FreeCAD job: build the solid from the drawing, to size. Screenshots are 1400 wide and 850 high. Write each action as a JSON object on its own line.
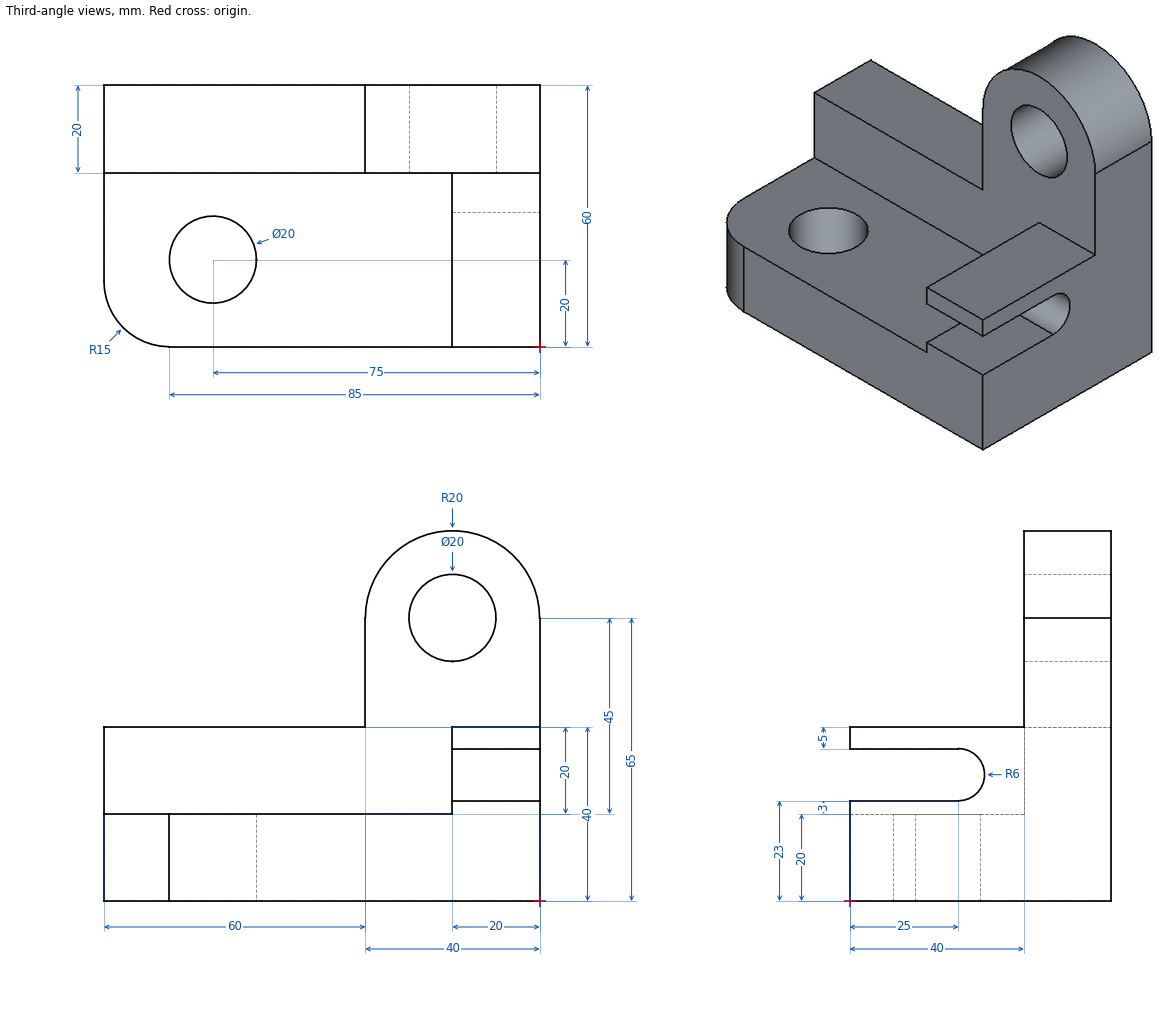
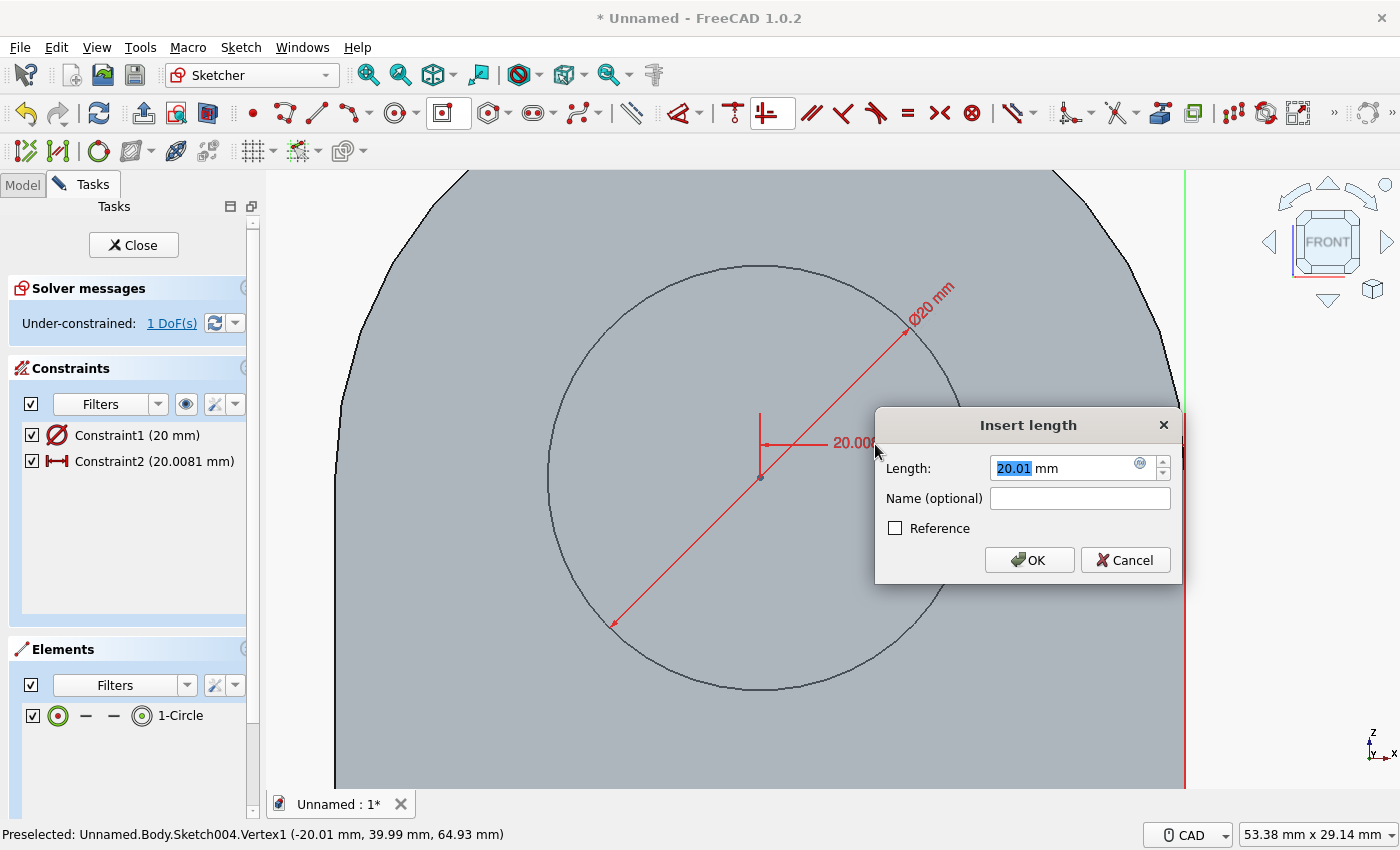
{"action": "type", "text": "20"}
{"action": "key", "text": "Return"}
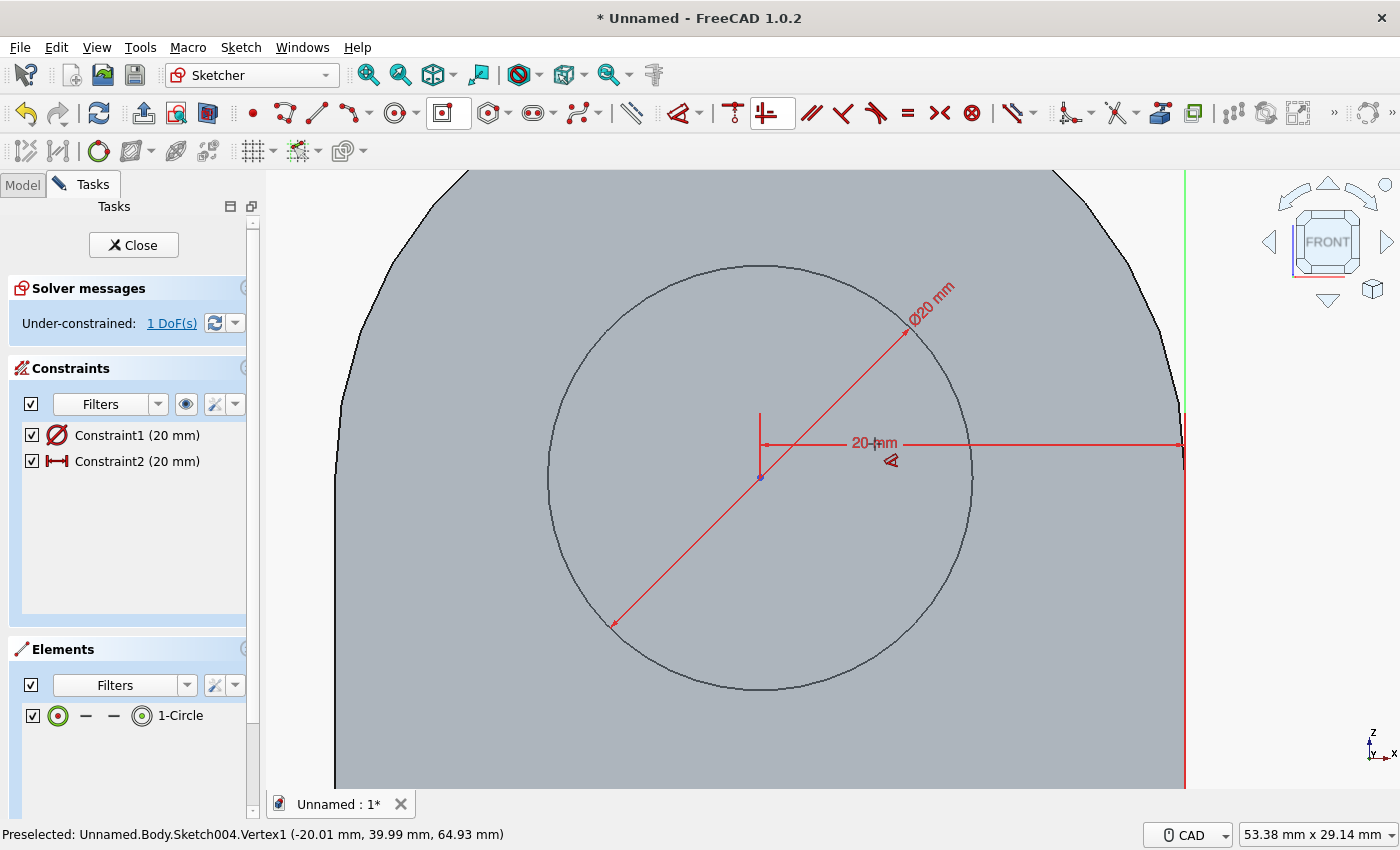
{"action": "left_click", "coordinate": [760, 478]}
{"action": "left_click", "coordinate": [1219, 620]}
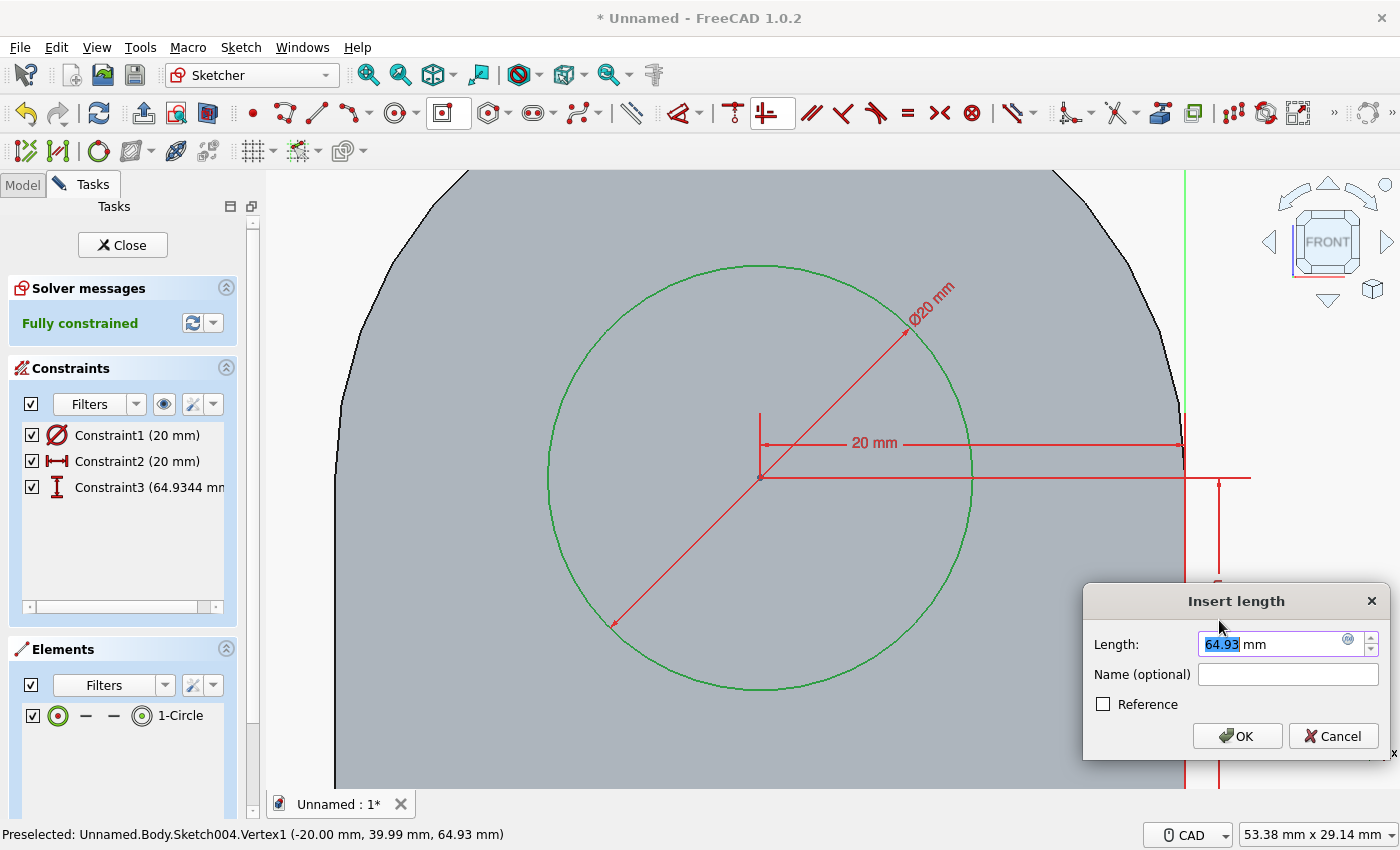
{"action": "type", "text": "65"}
{"action": "key", "text": "Return"}
{"action": "key", "text": "Escape"}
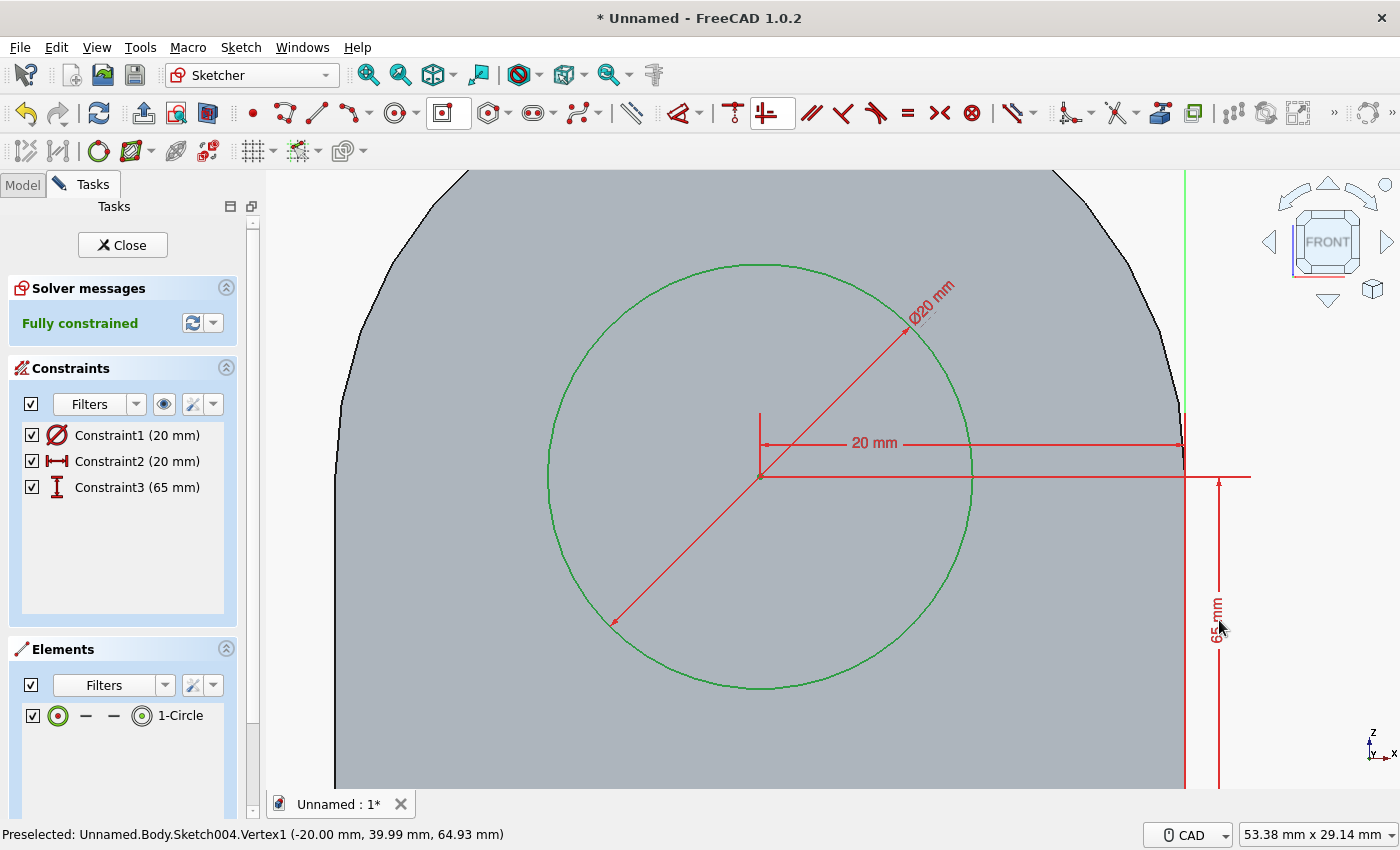
{"action": "left_click", "coordinate": [123, 245]}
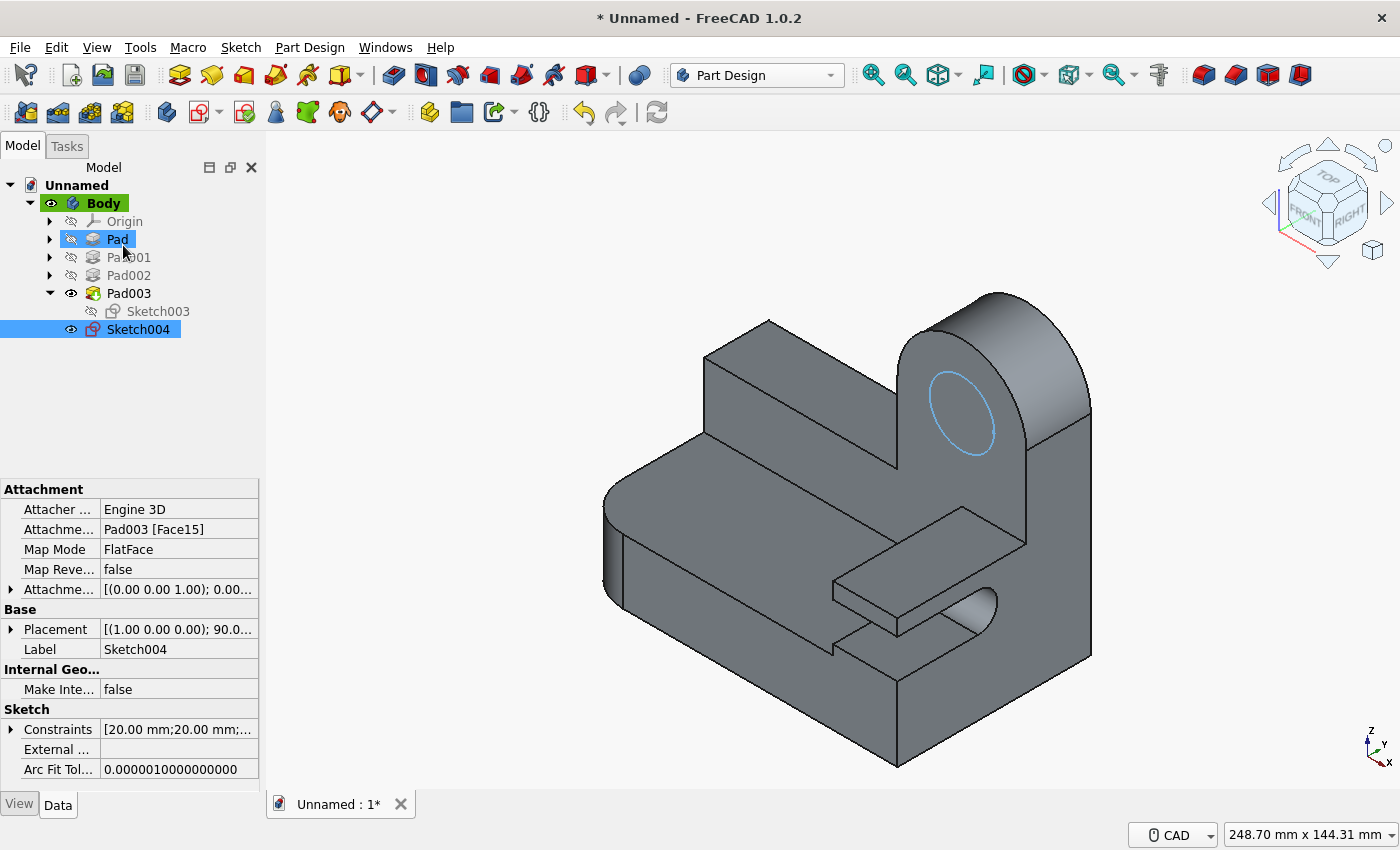
{"action": "left_click", "coordinate": [394, 76]}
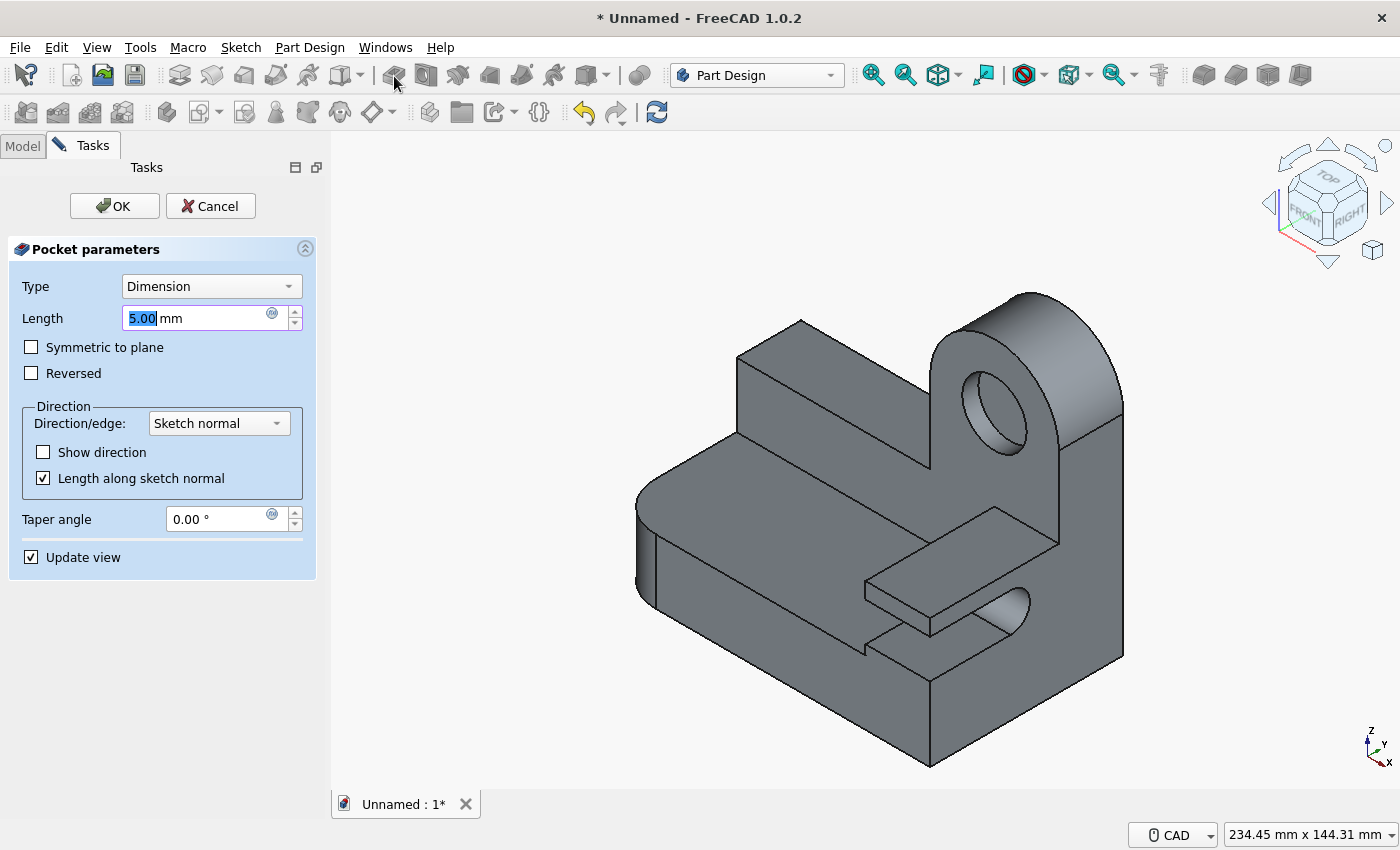
{"action": "type", "text": "20"}
{"action": "key", "text": "Tab"}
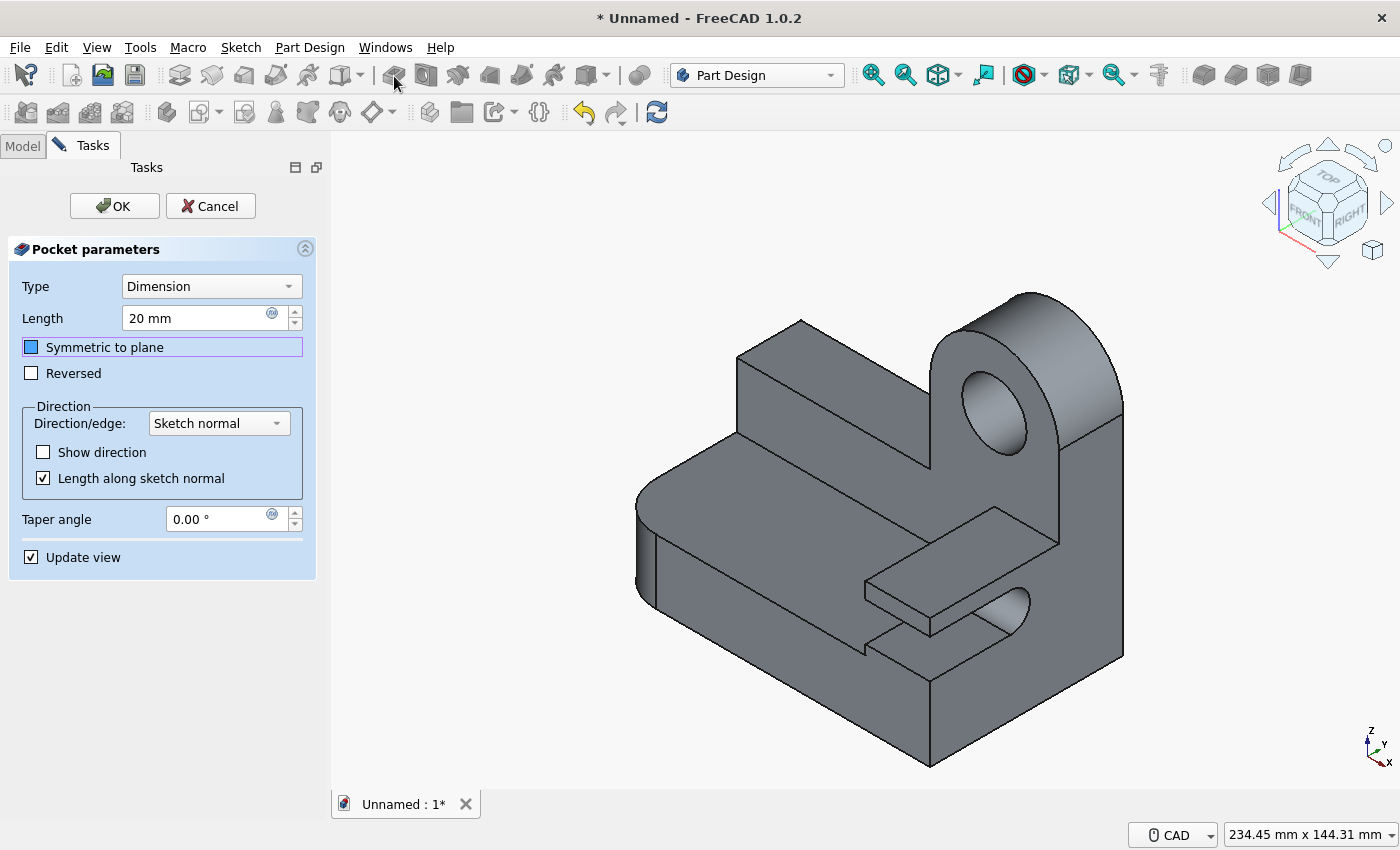
{"action": "left_click", "coordinate": [115, 206]}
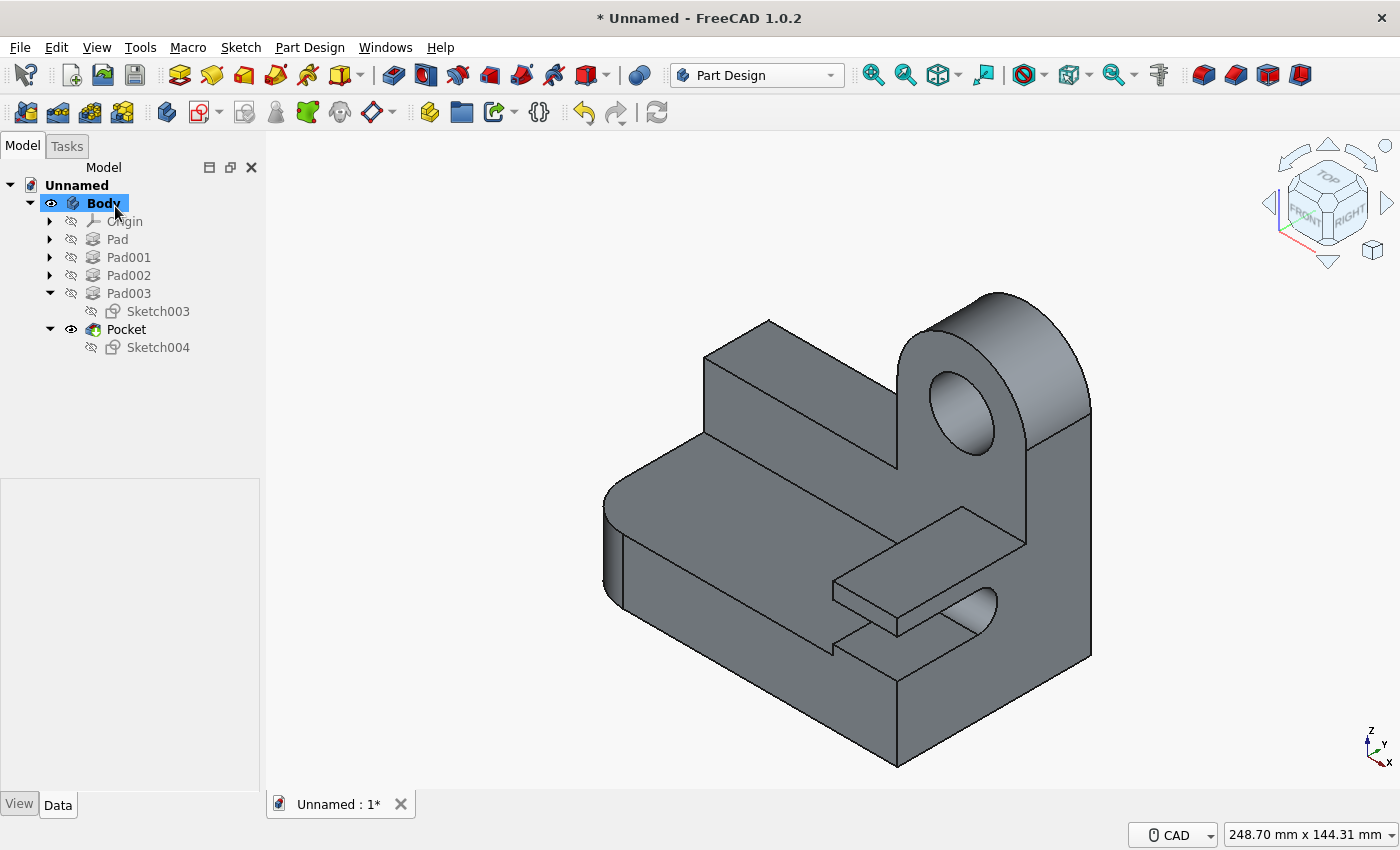
{"action": "left_click", "coordinate": [805, 564]}